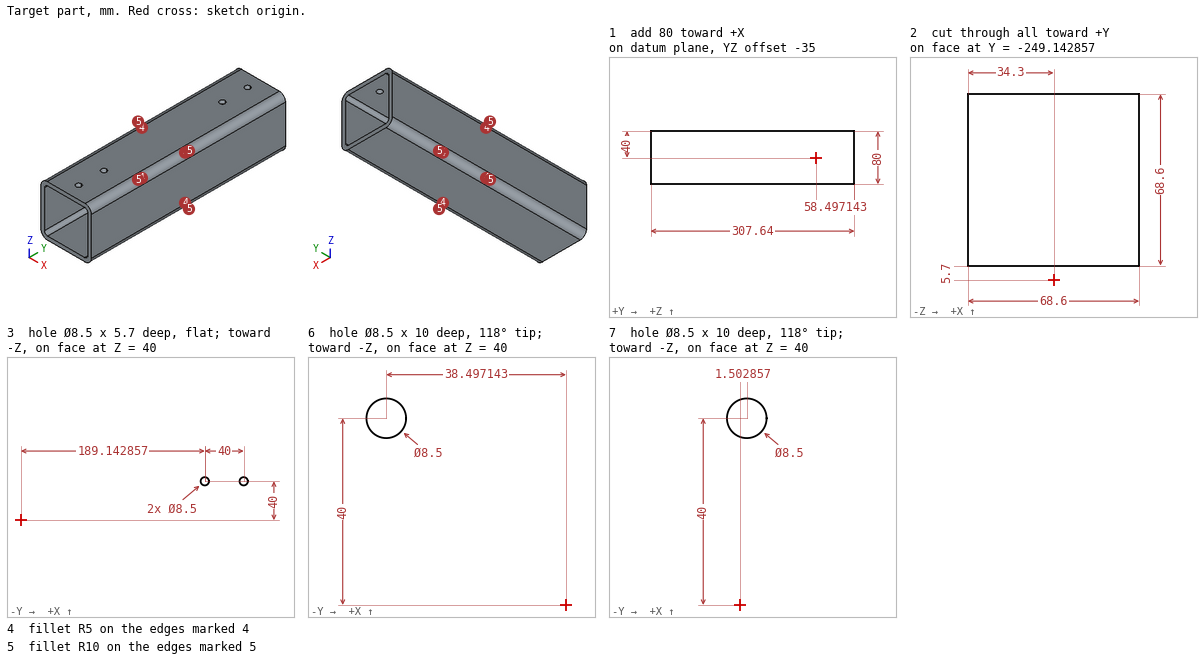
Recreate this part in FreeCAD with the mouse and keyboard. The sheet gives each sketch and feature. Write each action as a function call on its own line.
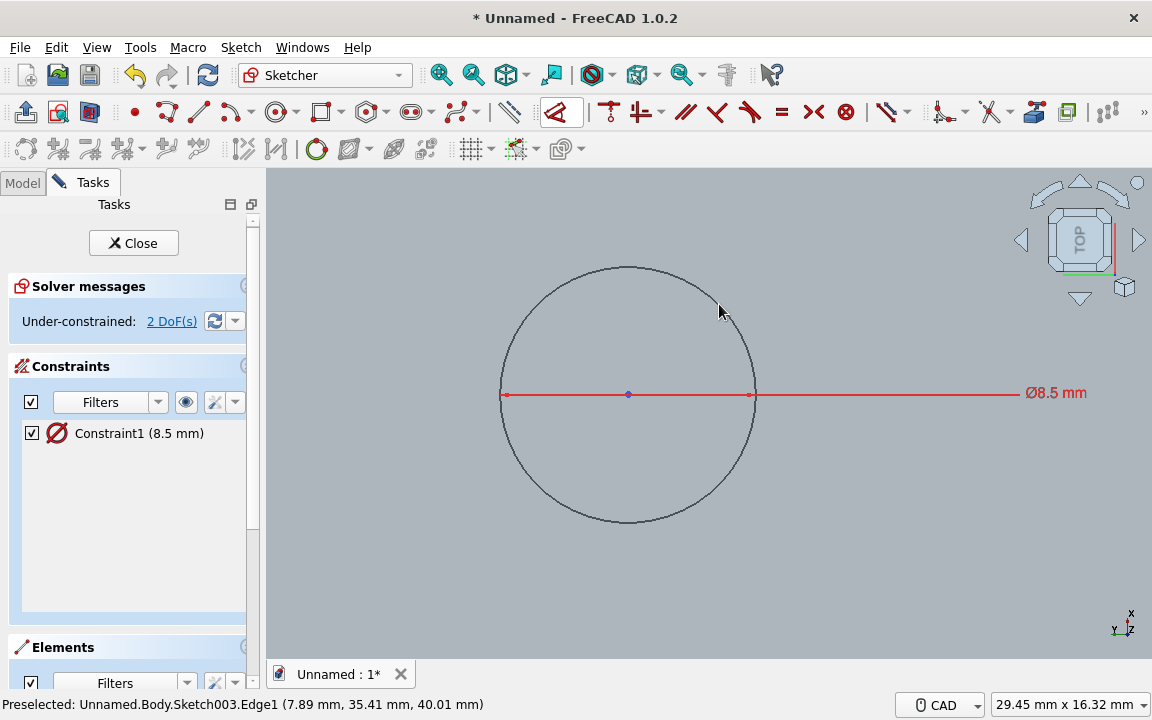
click(628, 395)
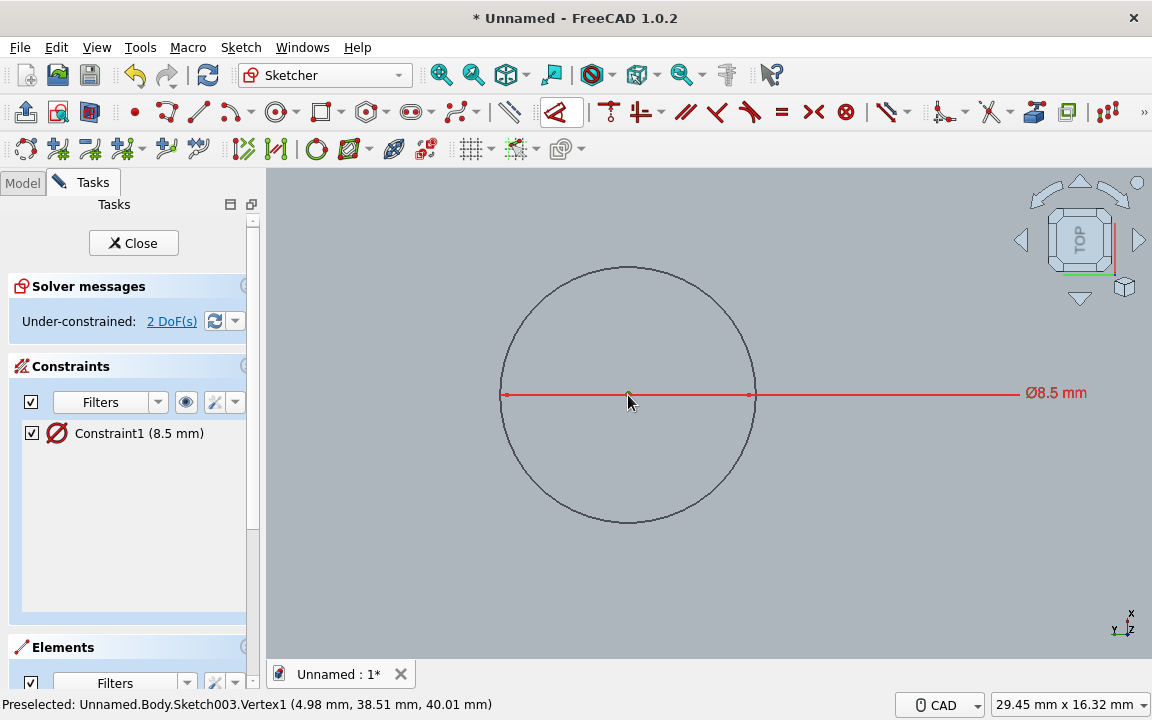
key(i)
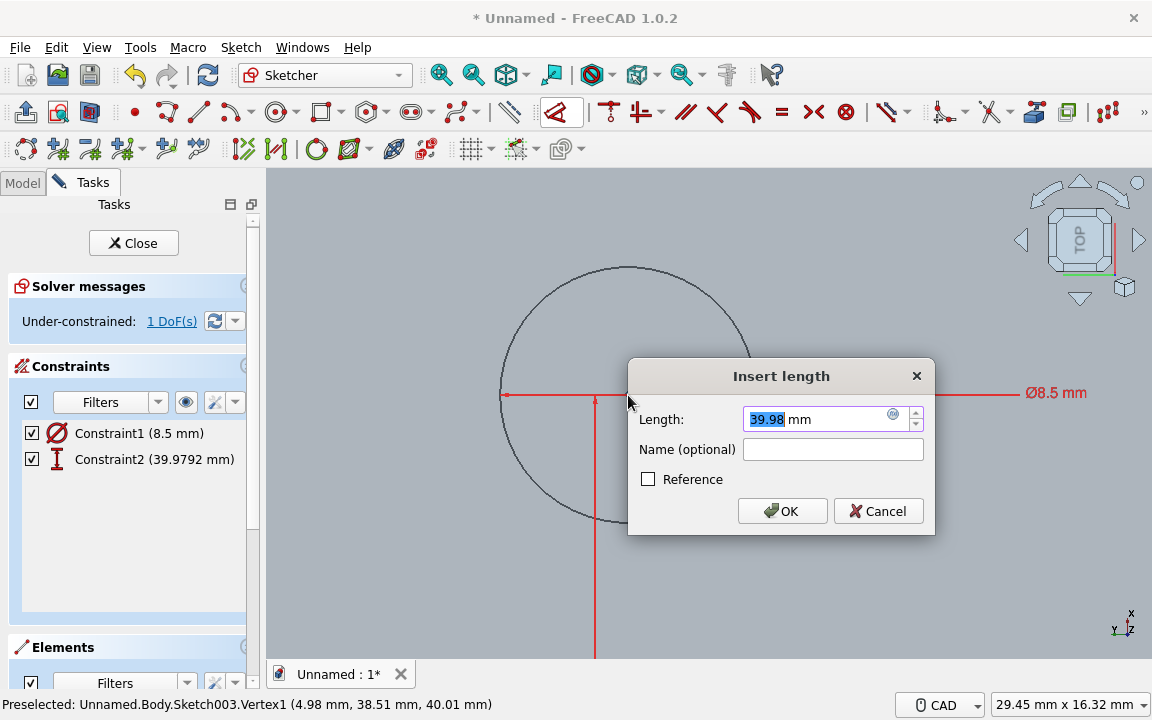
text(40)
key(Return)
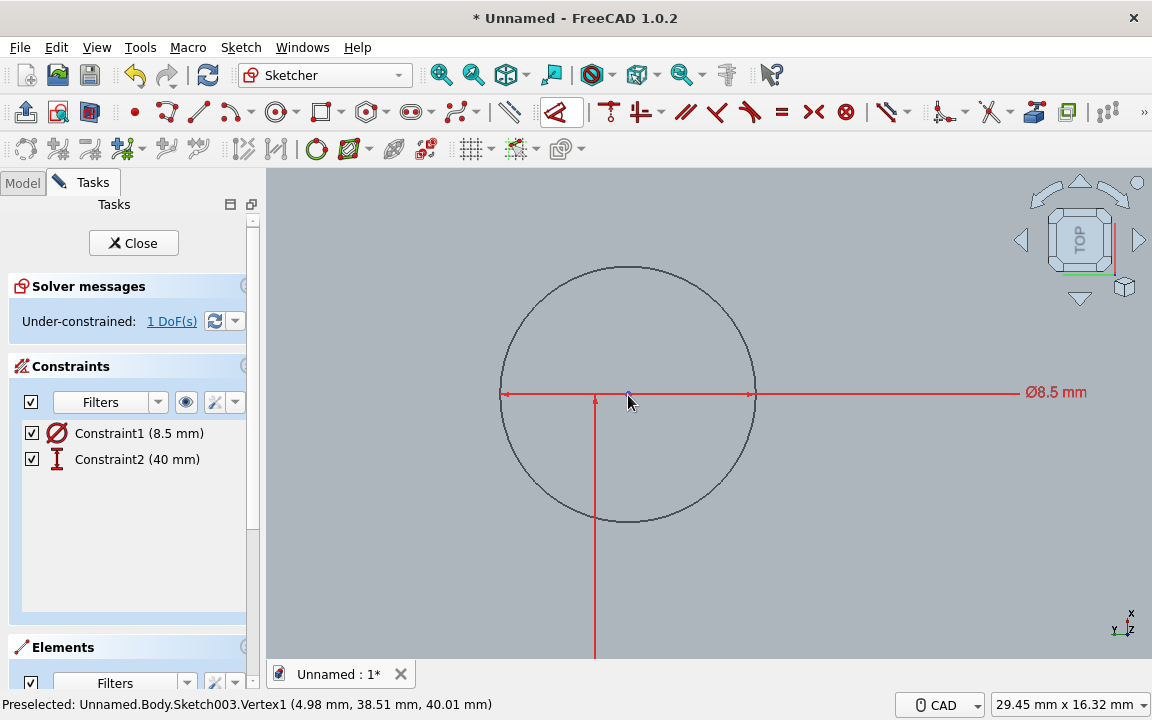
click(628, 394)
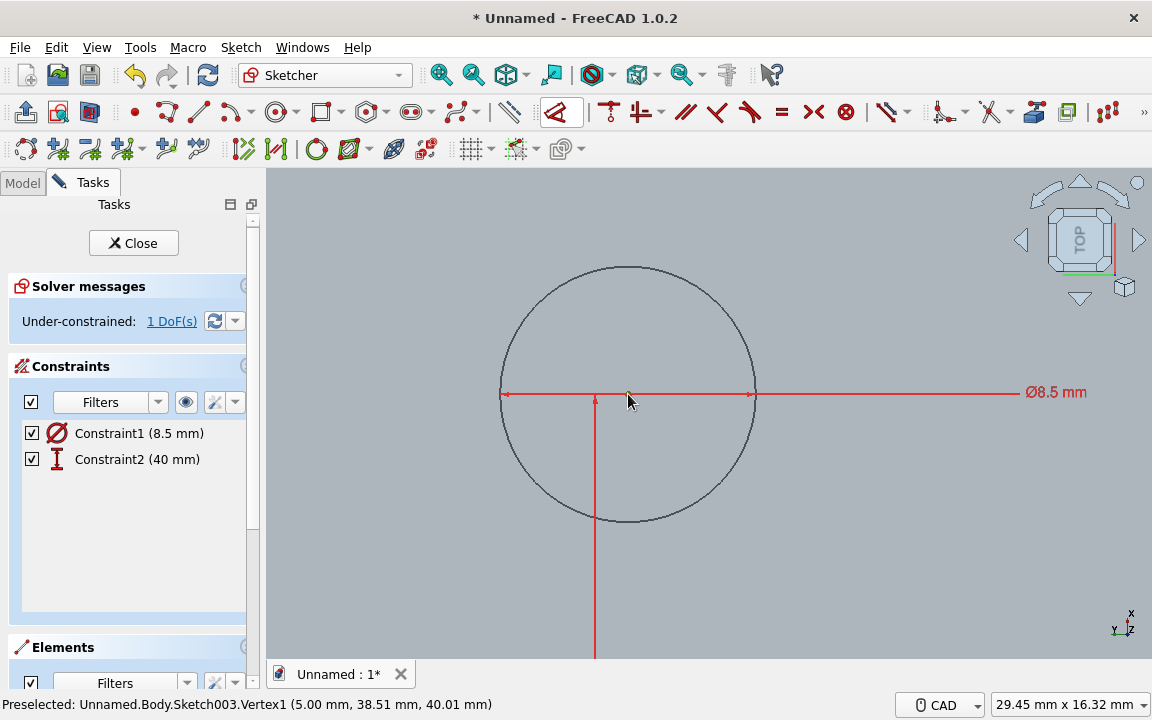
click(578, 112)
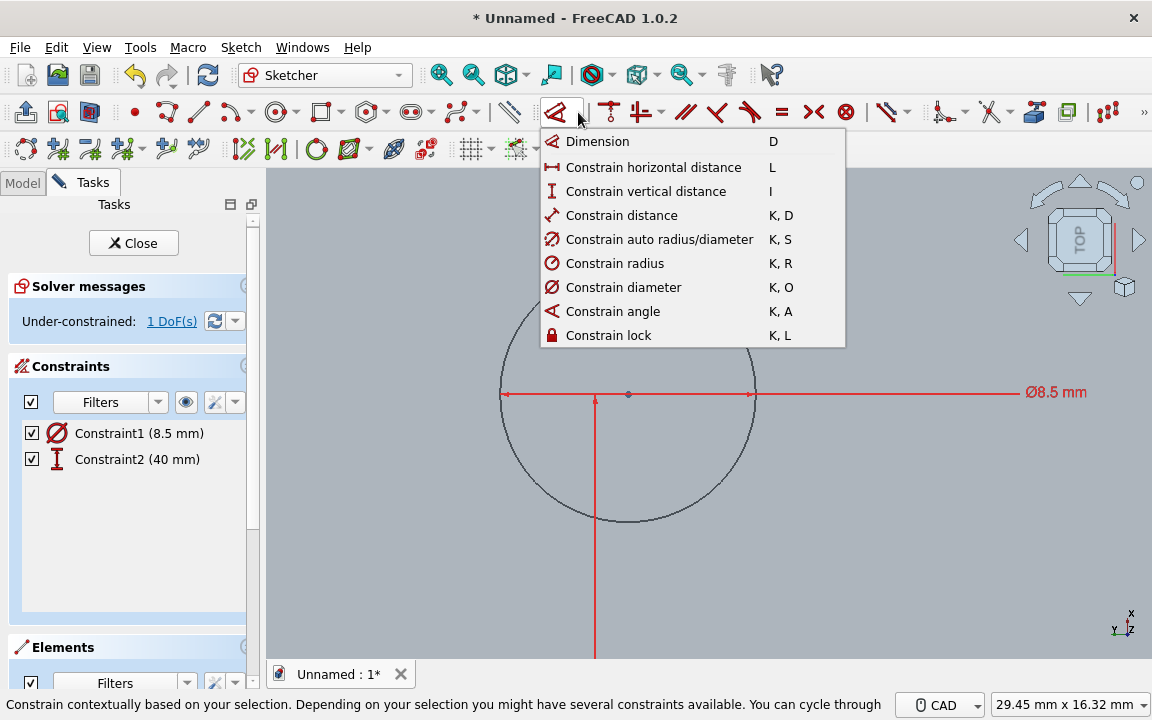
click(693, 167)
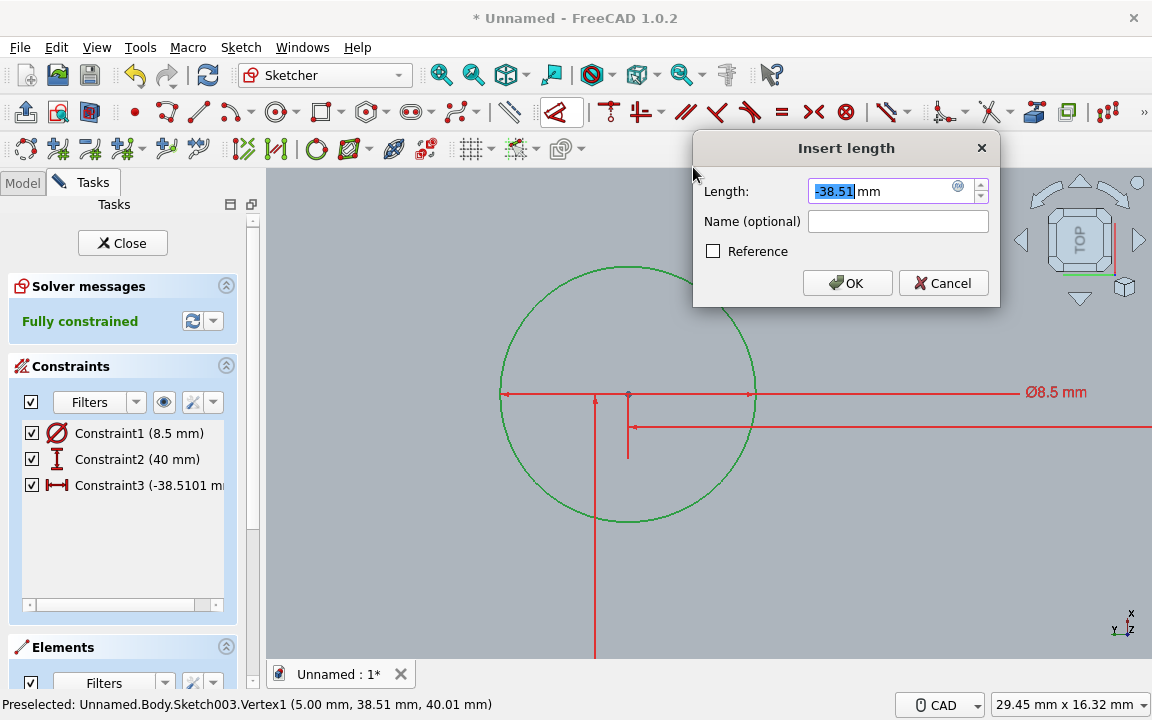
text(-38.497143)
key(Return)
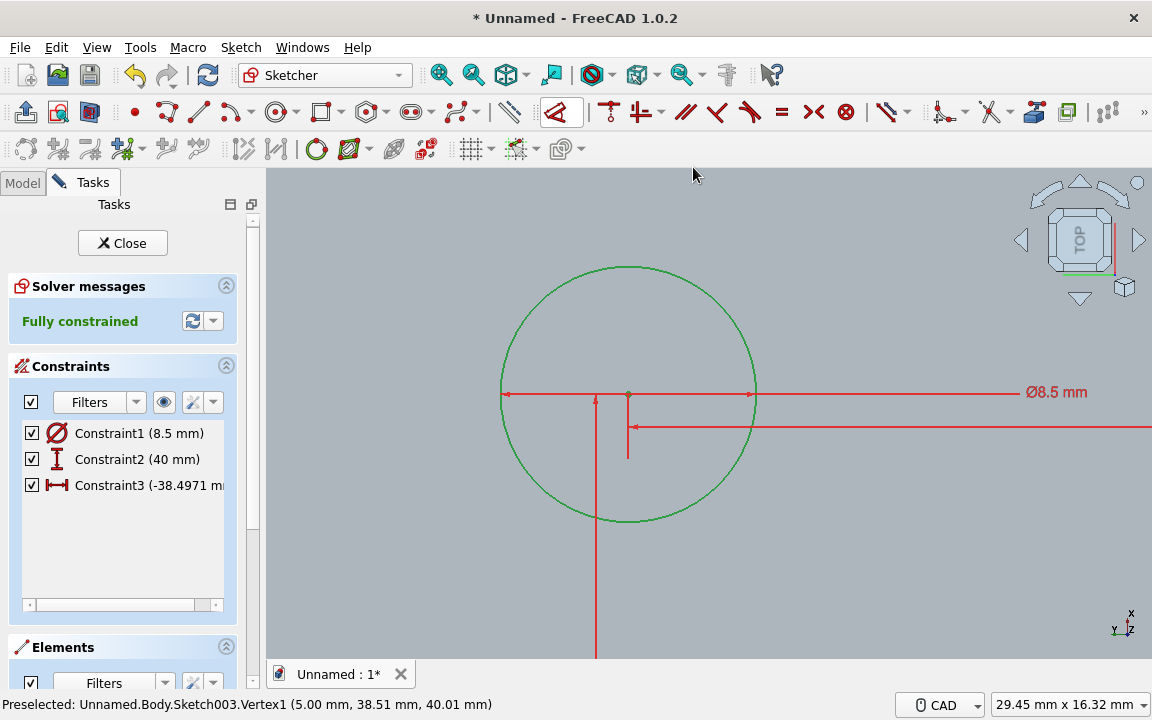
click(123, 243)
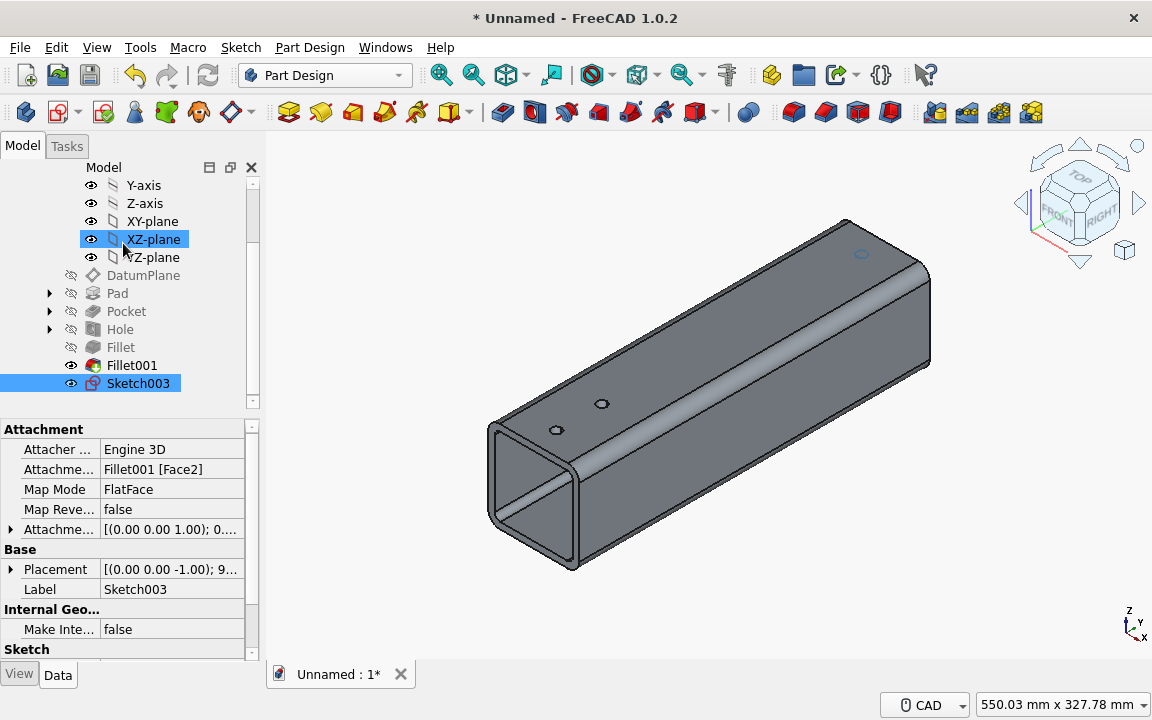
click(536, 112)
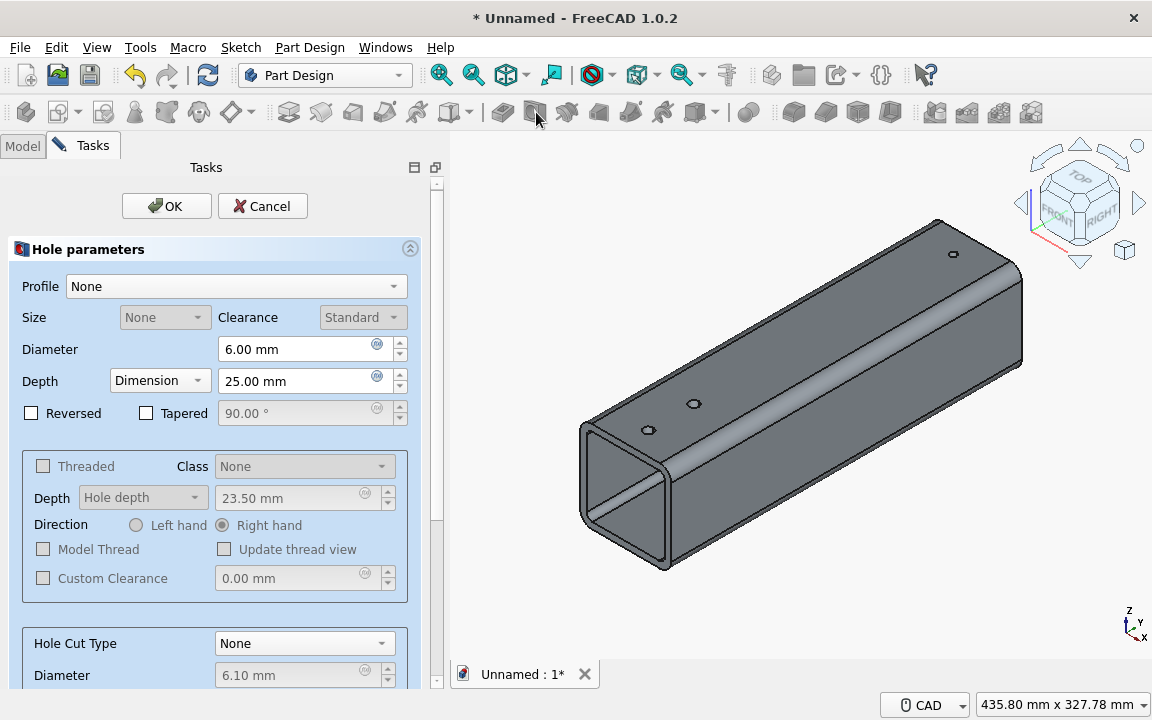
triple_click(305, 349)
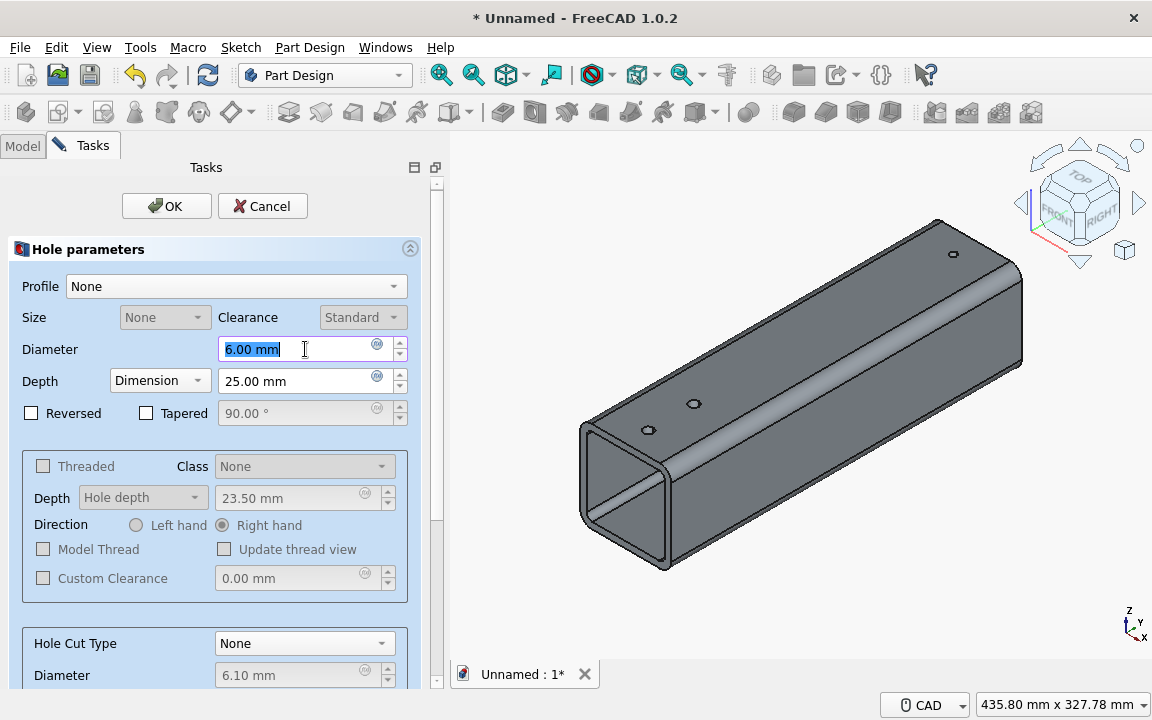
text(8.5)
key(Tab)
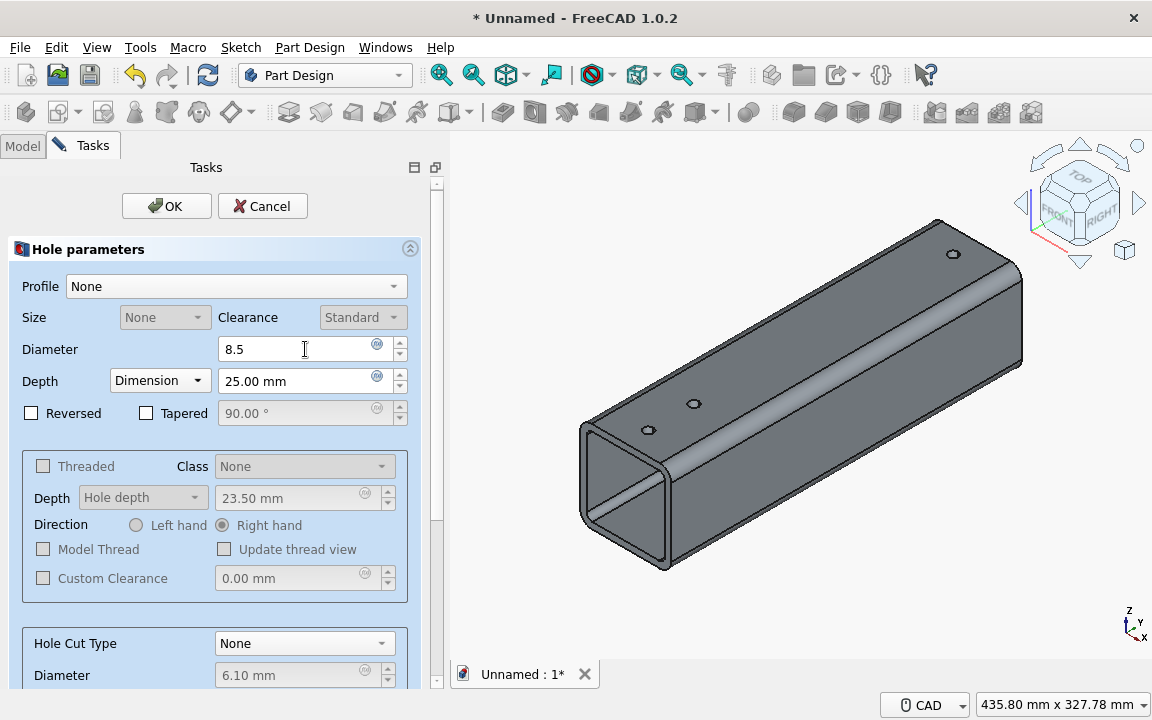
triple_click(305, 381)